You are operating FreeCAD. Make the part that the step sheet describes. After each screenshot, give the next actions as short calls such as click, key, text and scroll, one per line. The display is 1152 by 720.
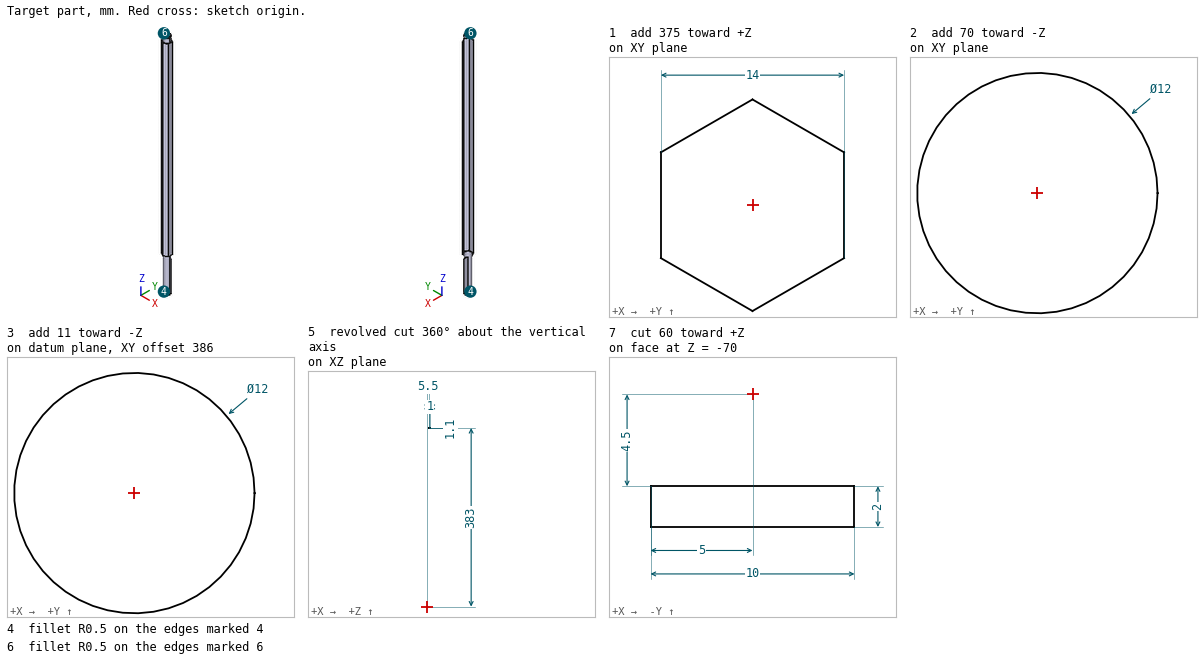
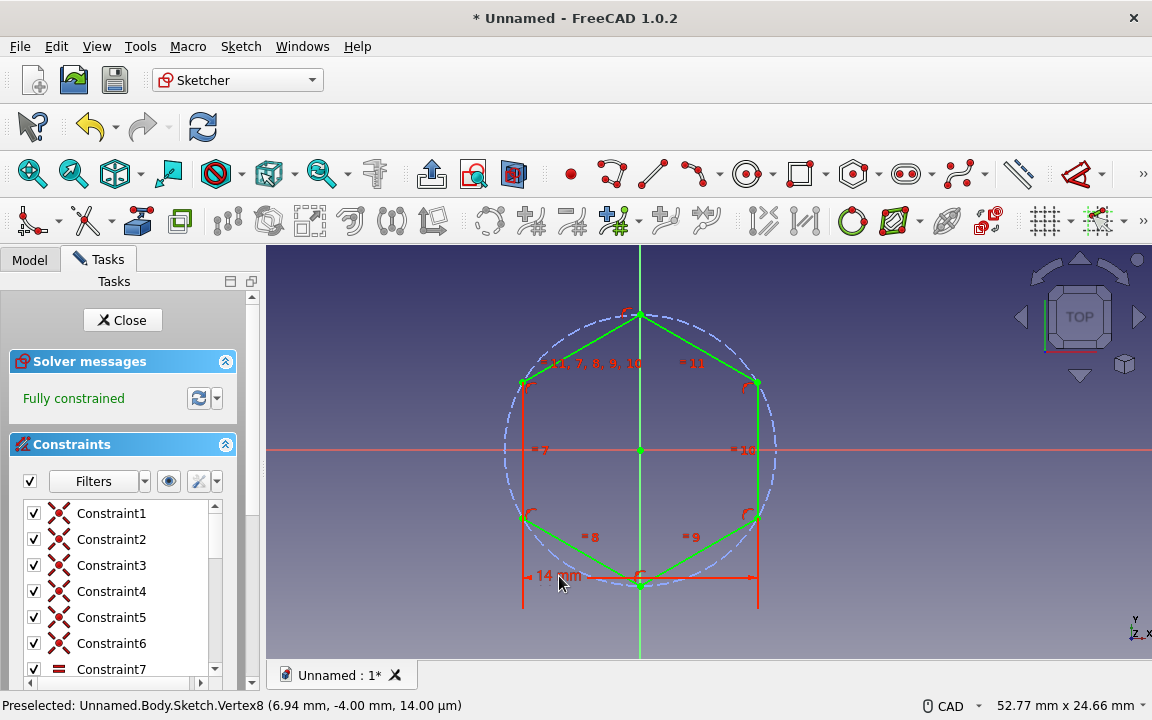
click(123, 320)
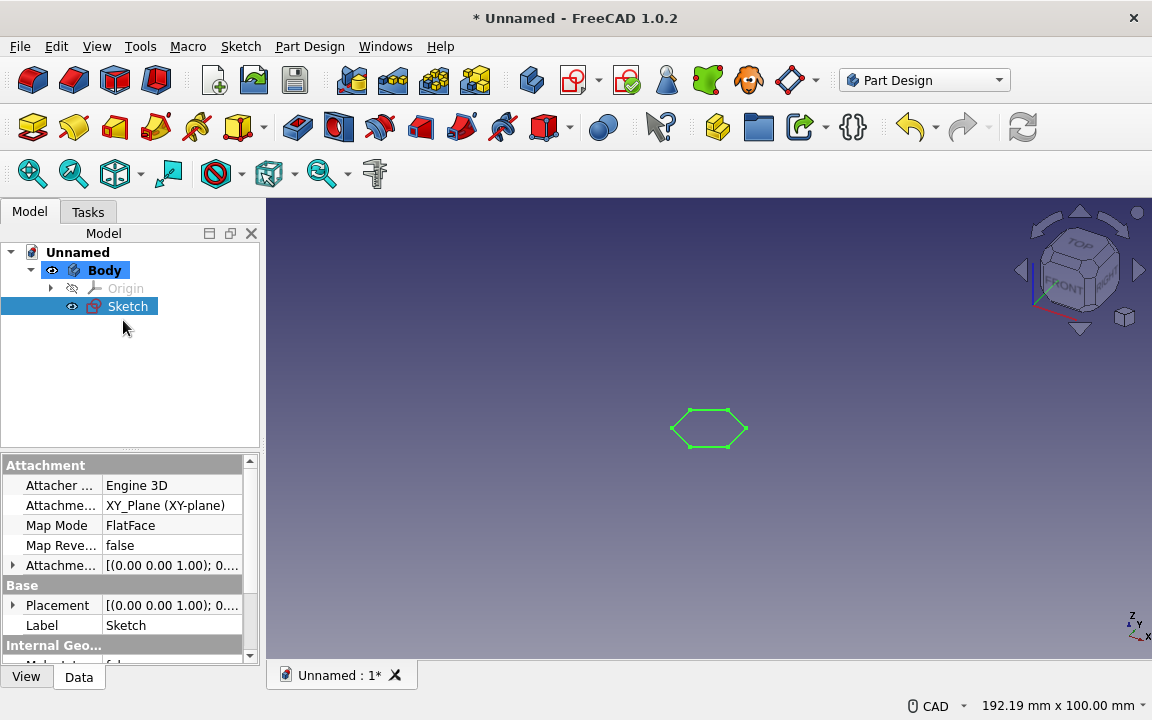
click(33, 128)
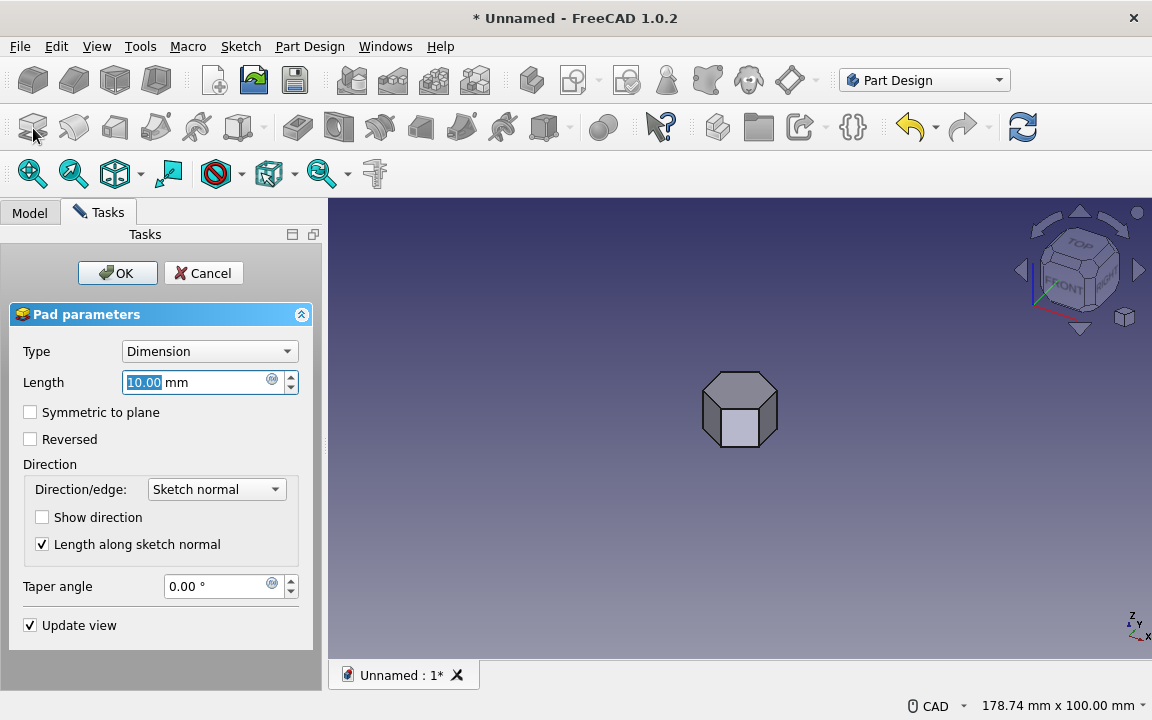
text(375)
key(Tab)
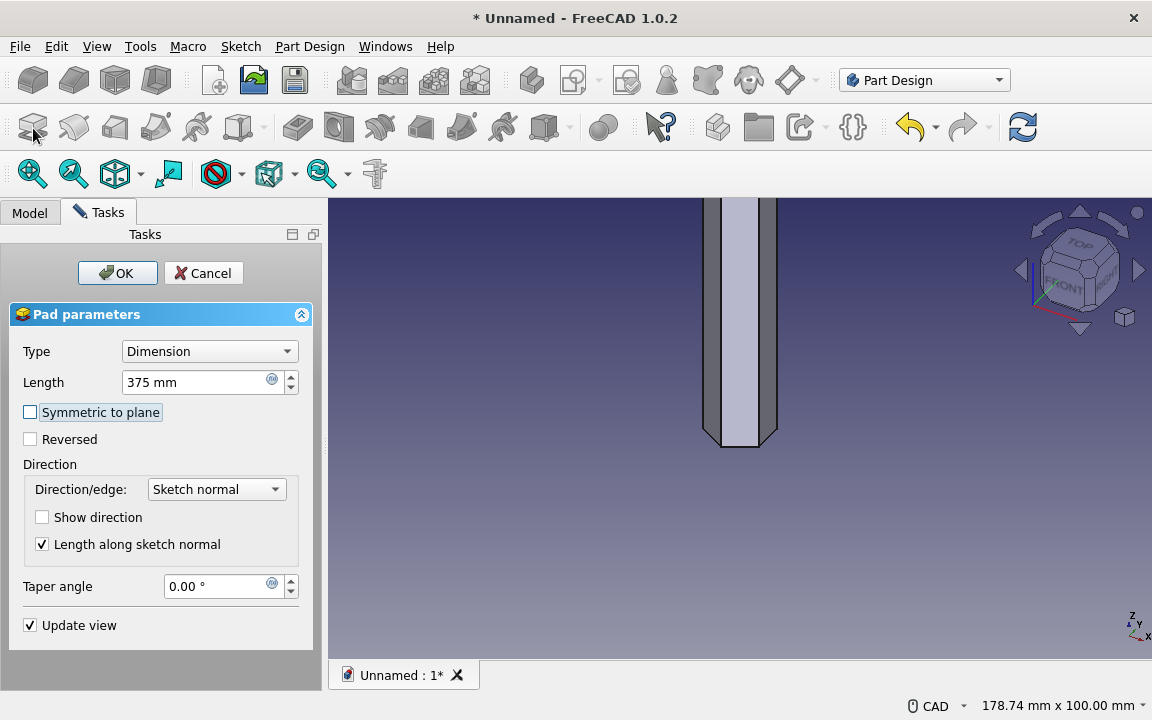
click(118, 273)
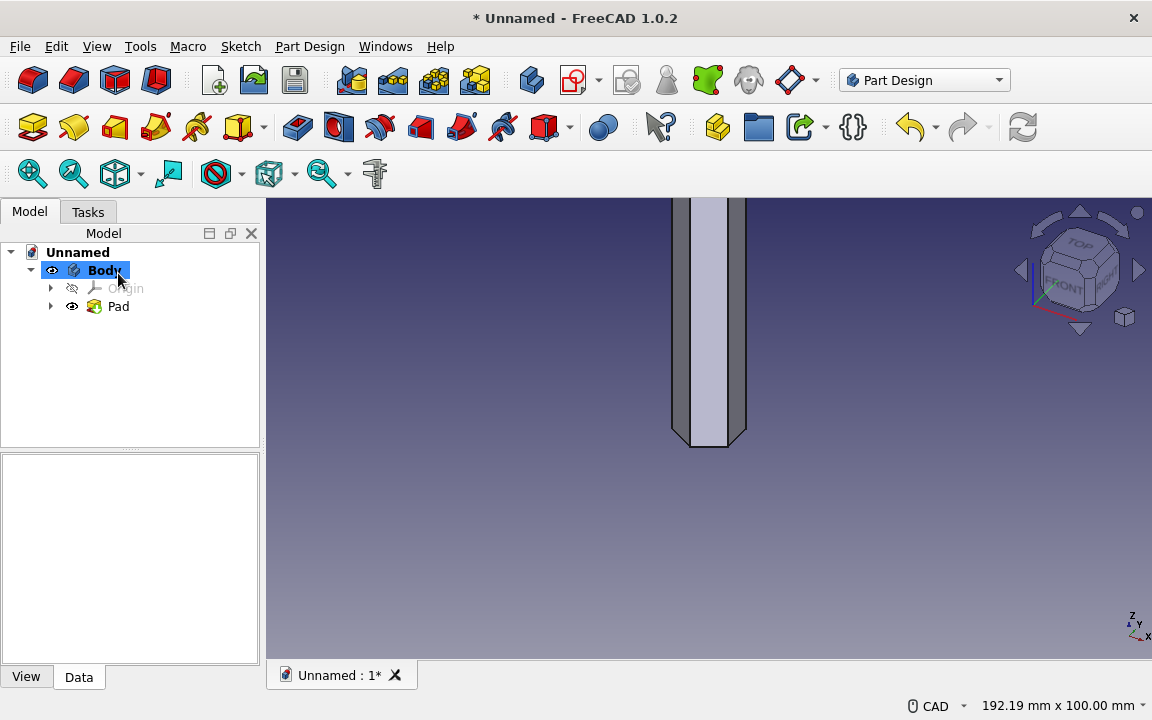
click(33, 174)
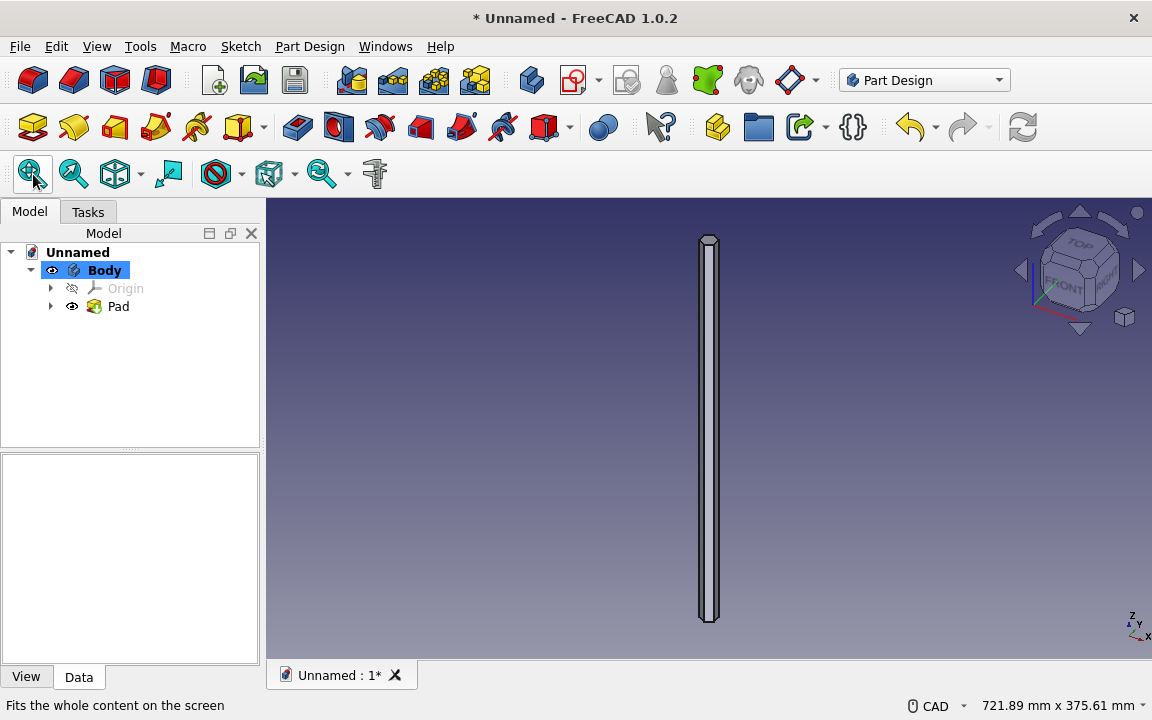
click(572, 80)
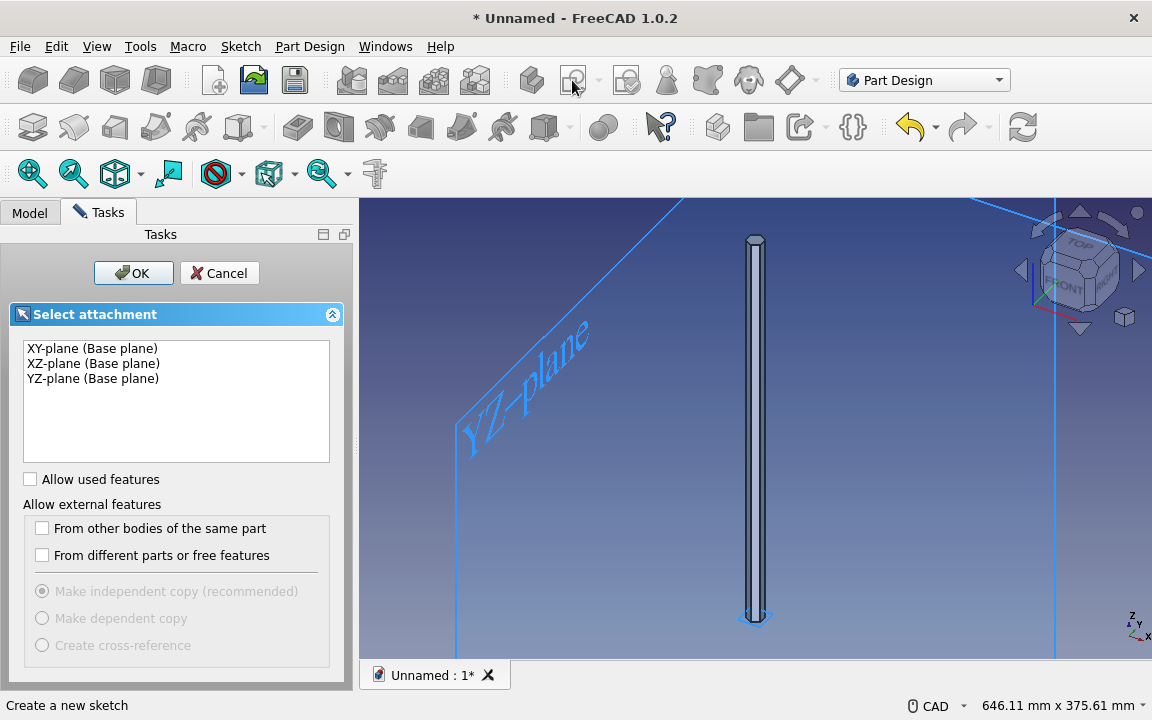
click(84, 348)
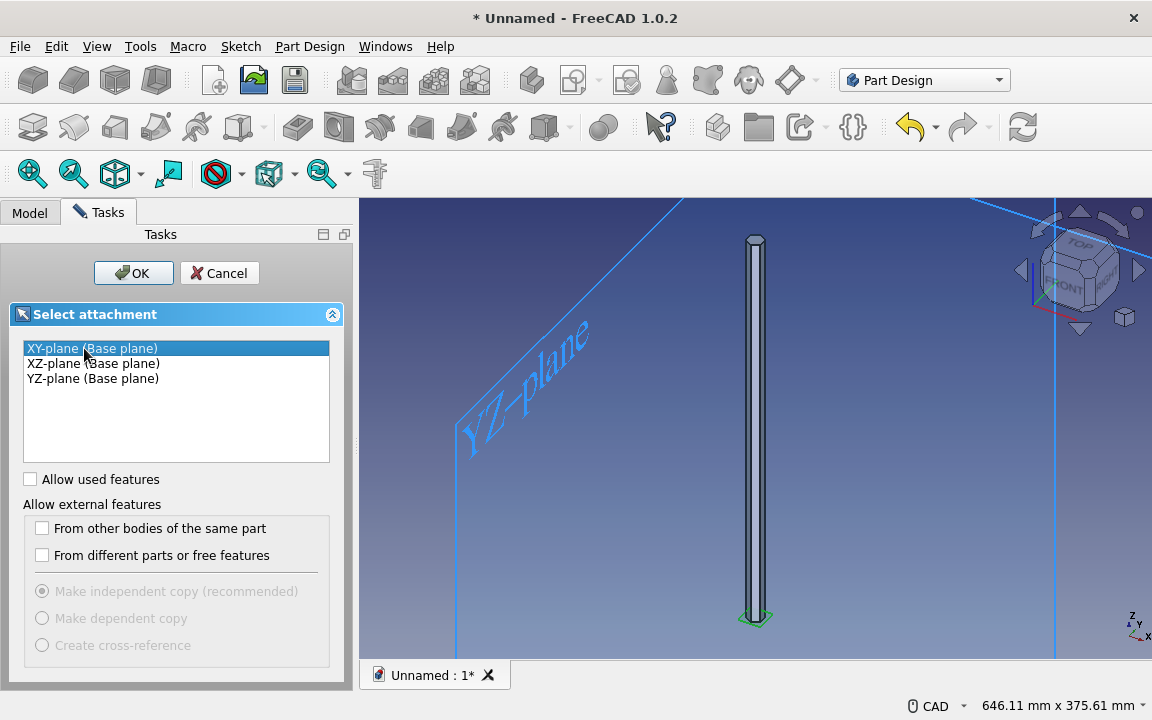
click(134, 273)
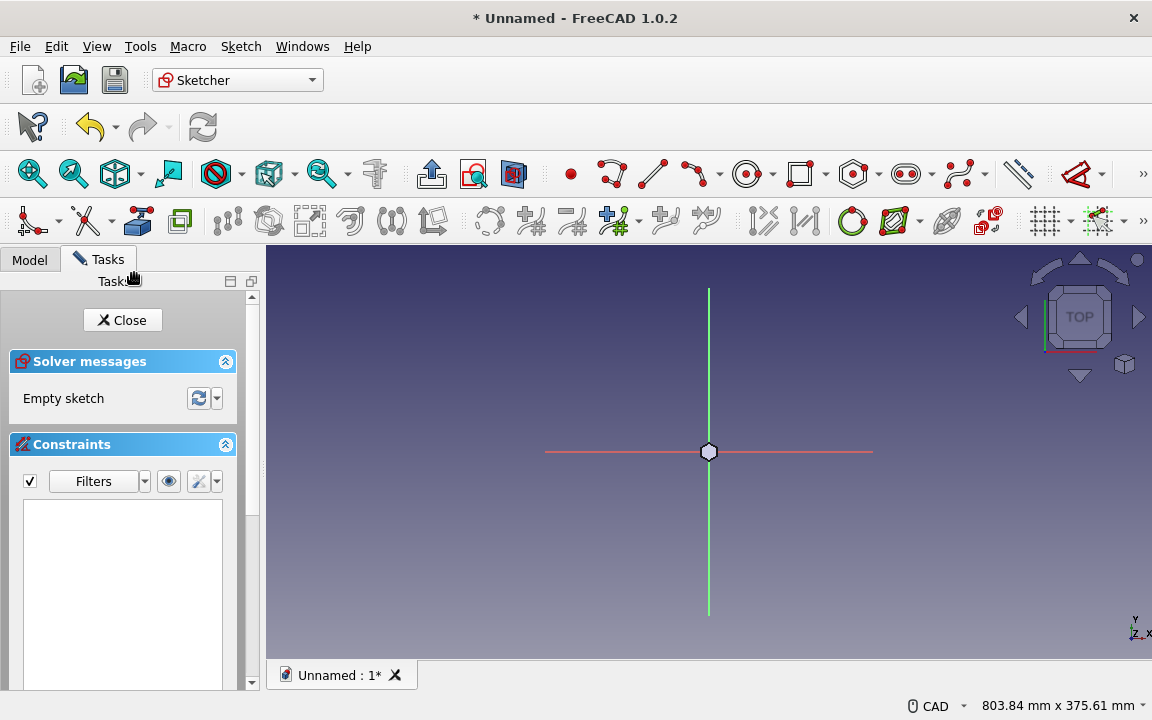
click(514, 174)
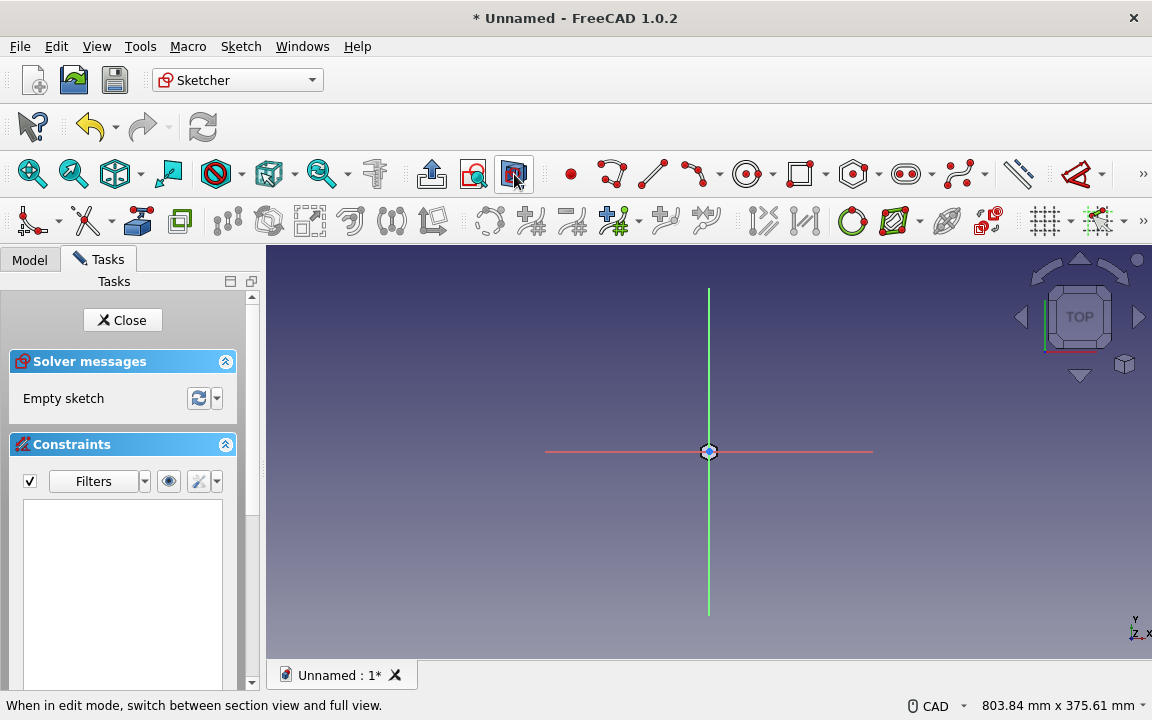
scroll(713, 452, up, 15)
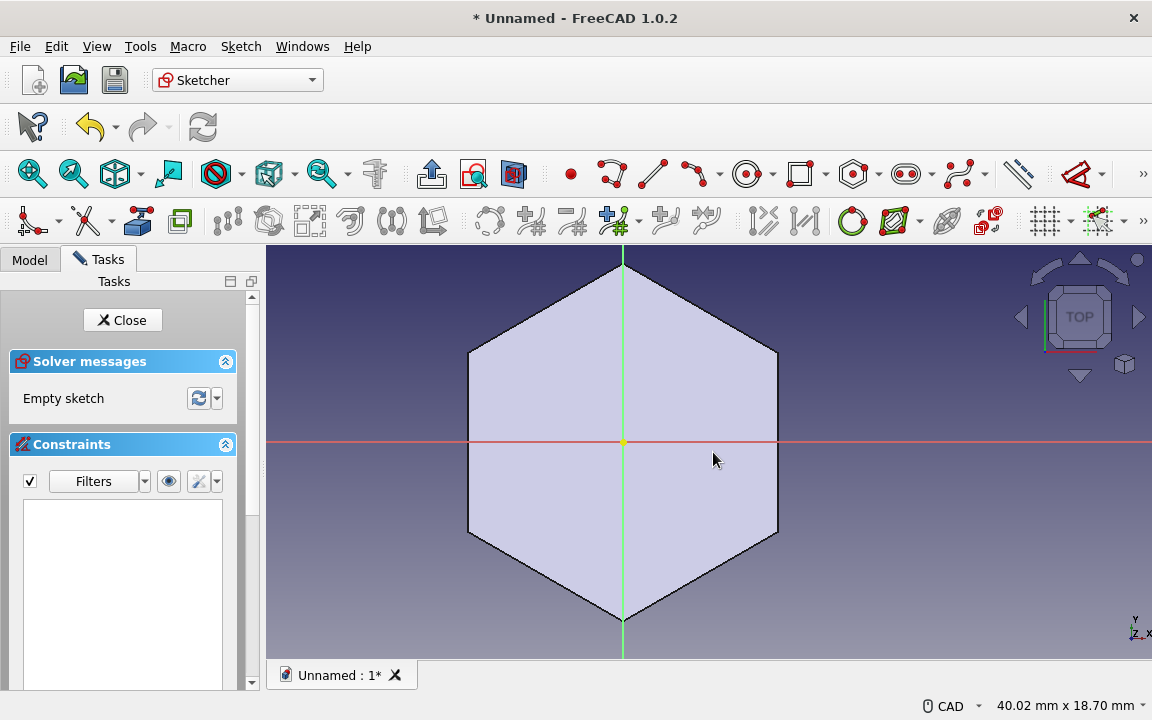
click(746, 174)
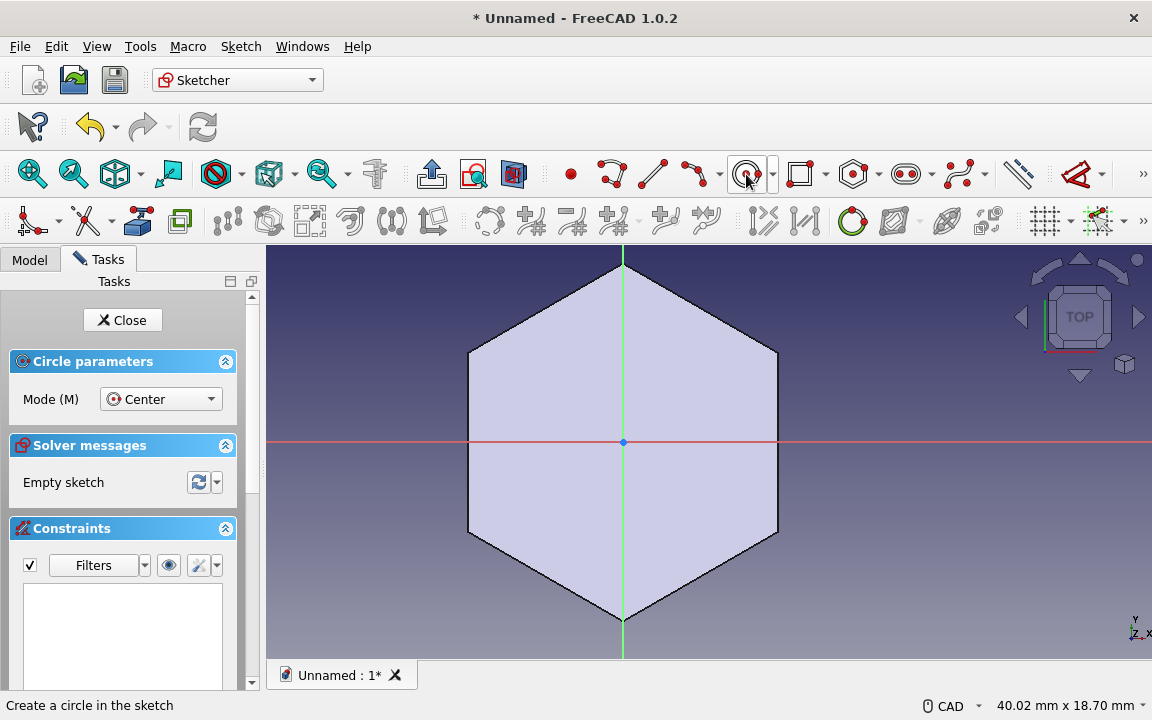
click(623, 442)
move(717, 349)